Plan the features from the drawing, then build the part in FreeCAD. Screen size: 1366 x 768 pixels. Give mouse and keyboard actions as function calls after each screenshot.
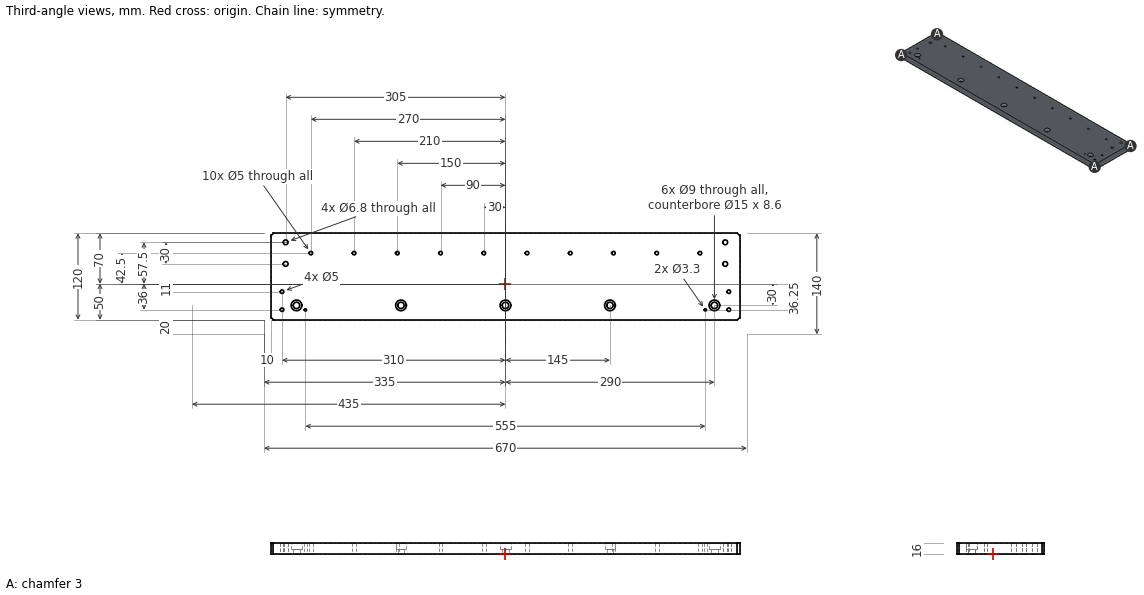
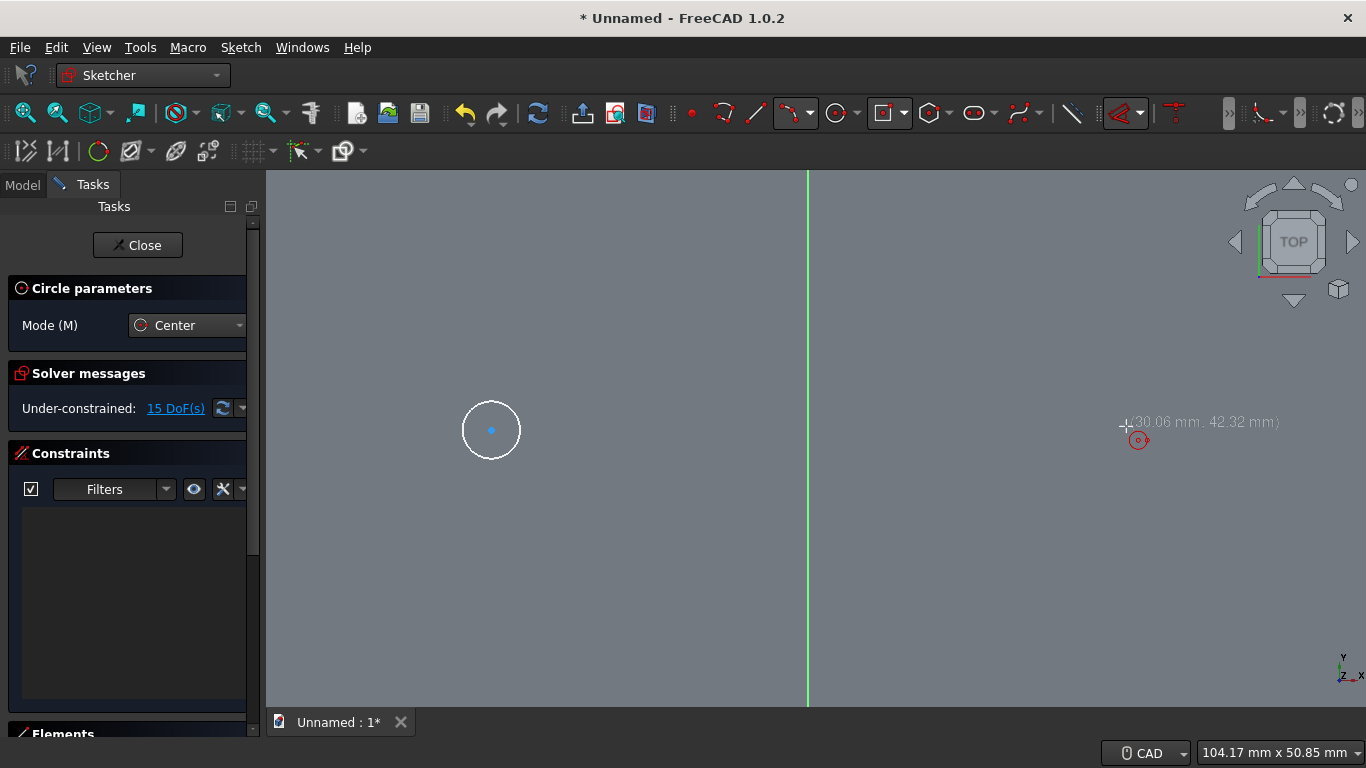
scroll(740, 414, down, 11)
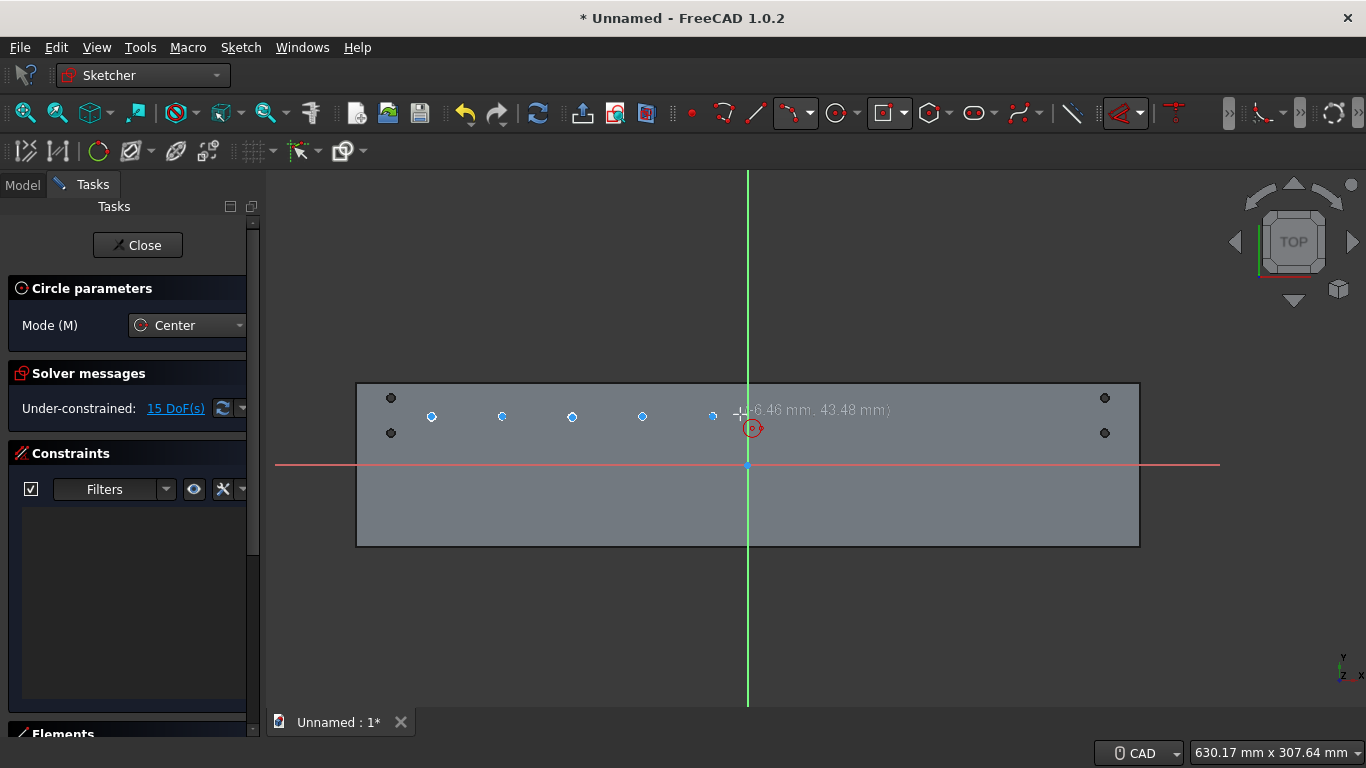
click(783, 416)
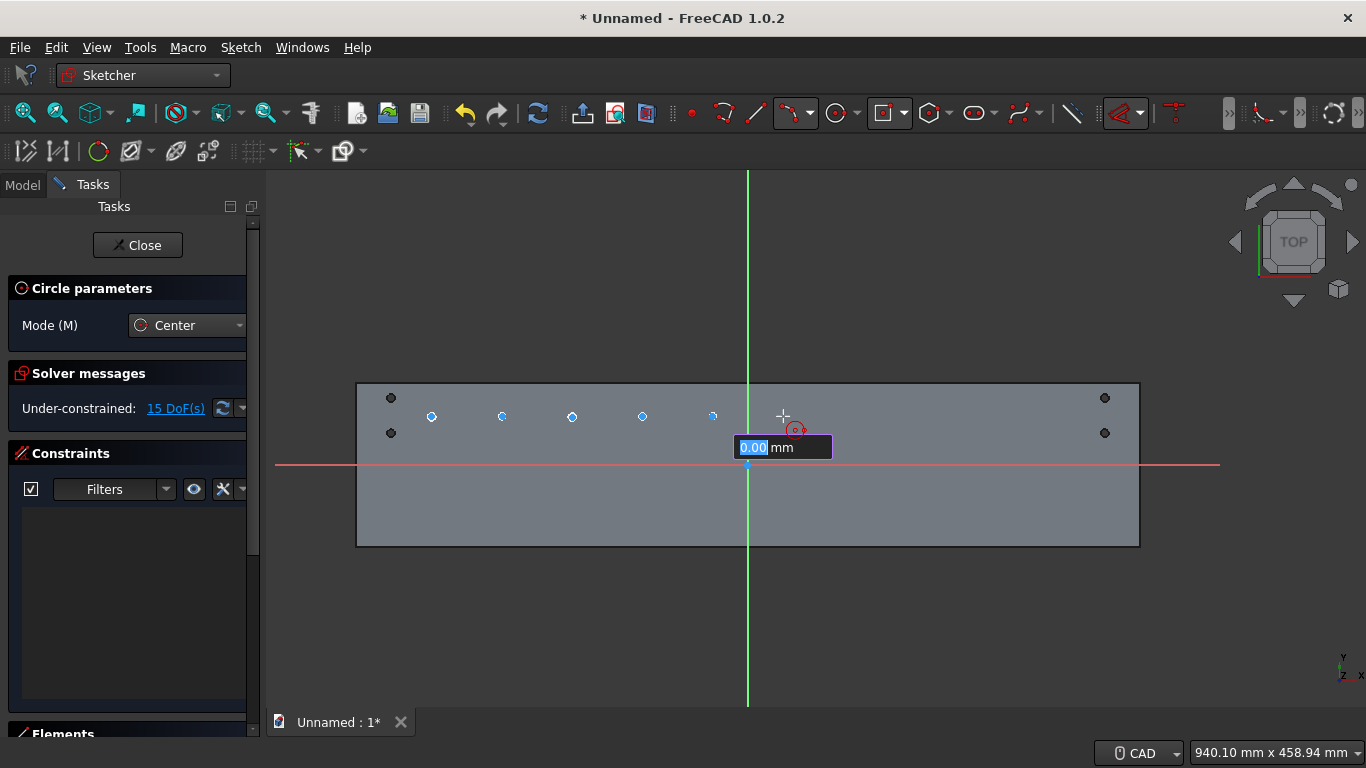
scroll(785, 414, up, 9)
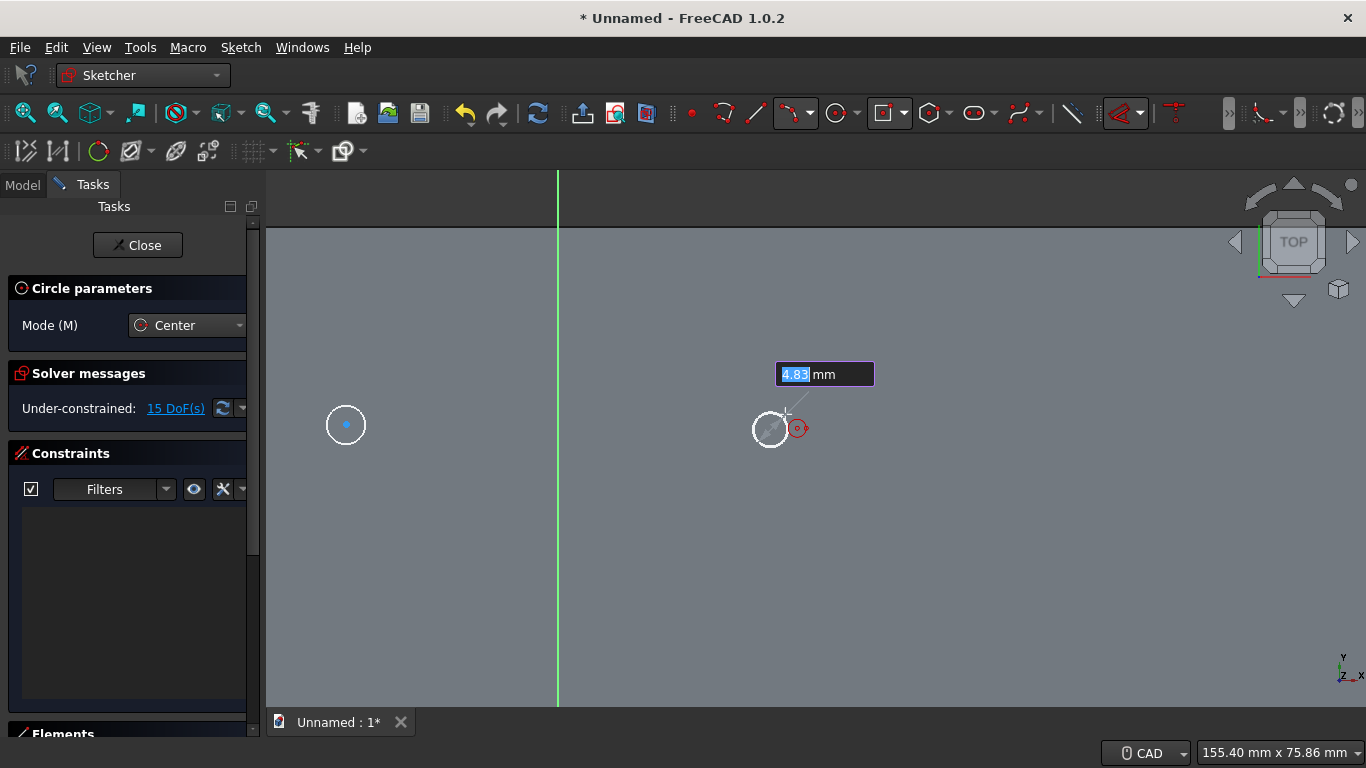
click(783, 409)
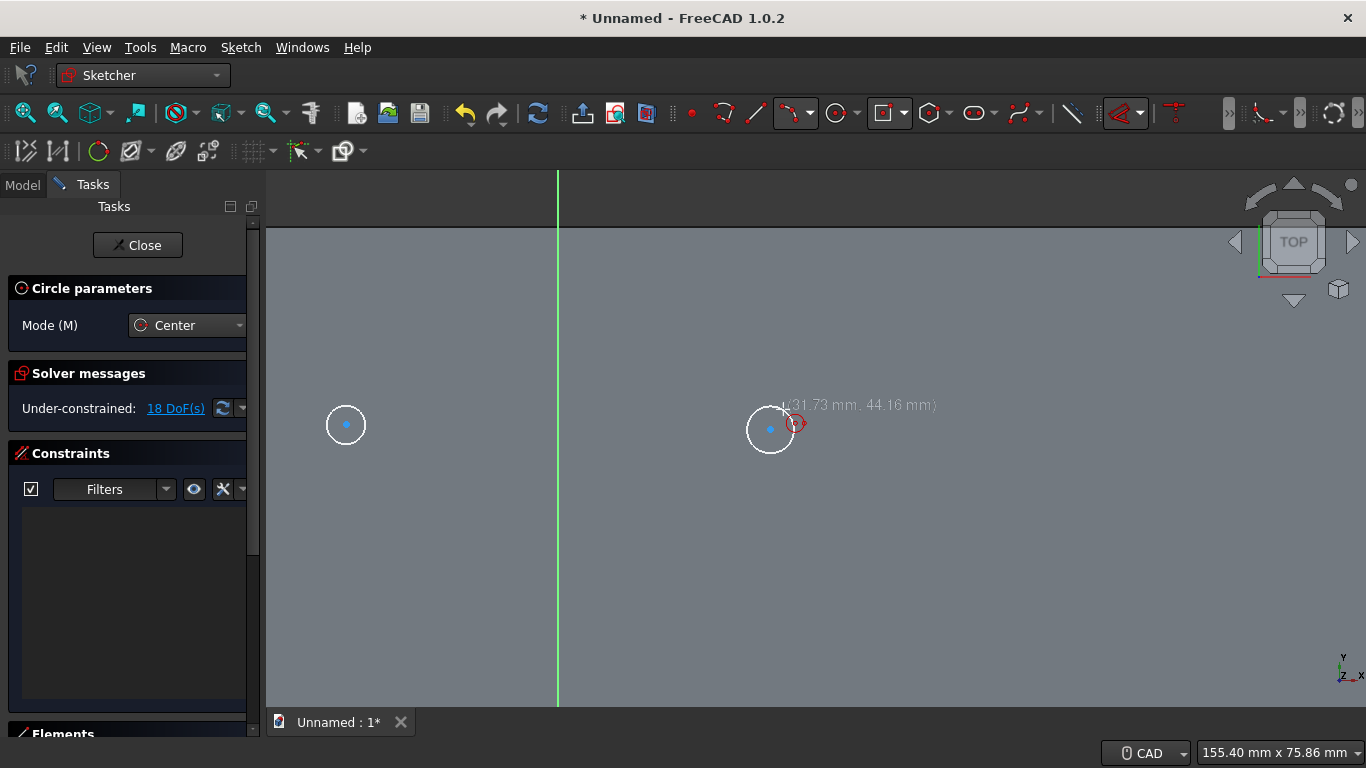
scroll(1195, 422, up, 2)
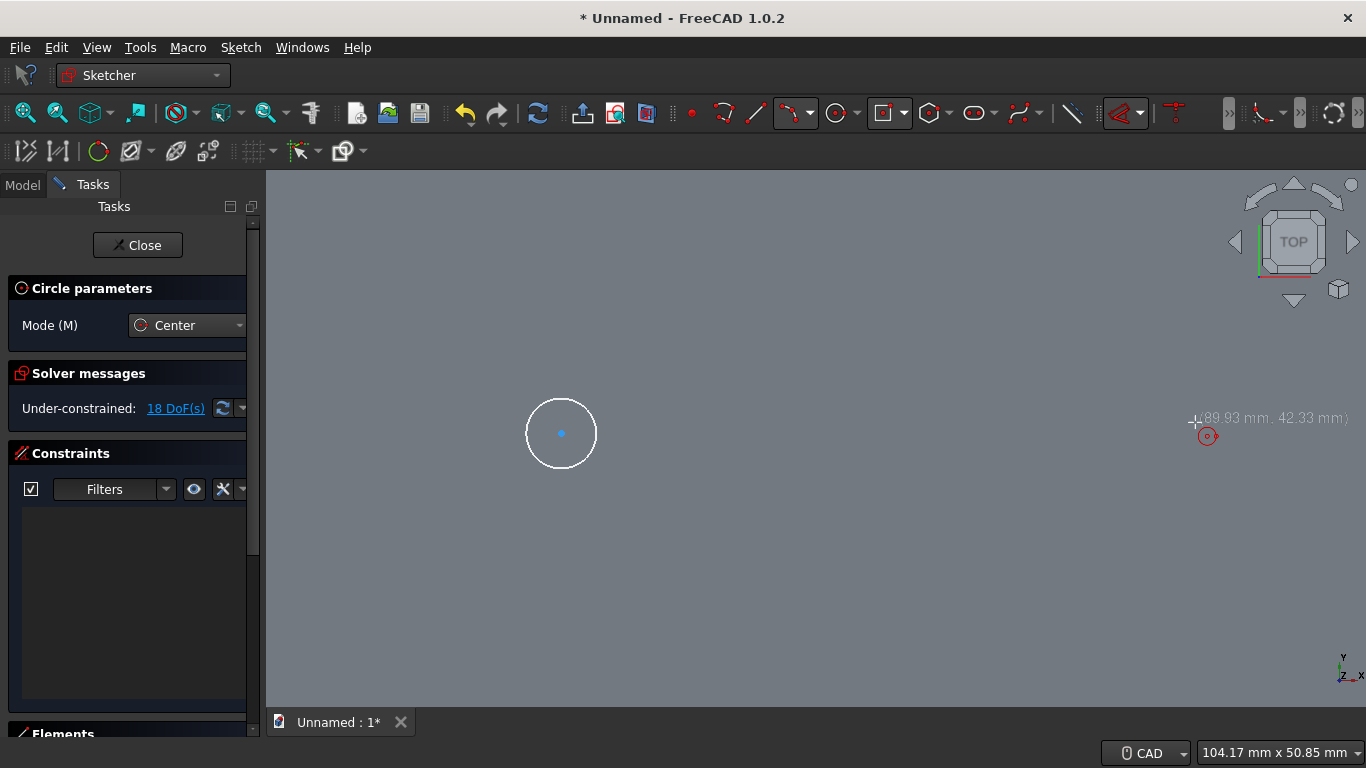
scroll(810, 414, down, 11)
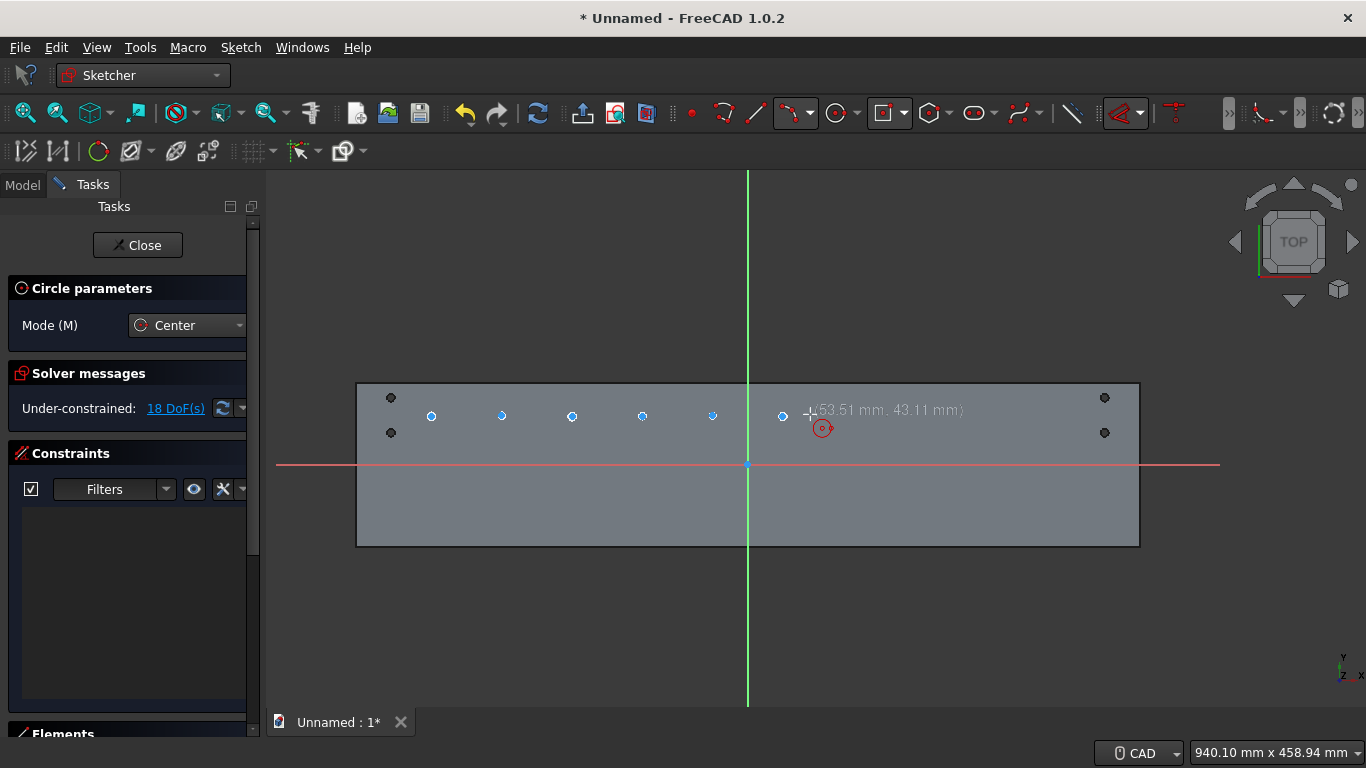
click(853, 415)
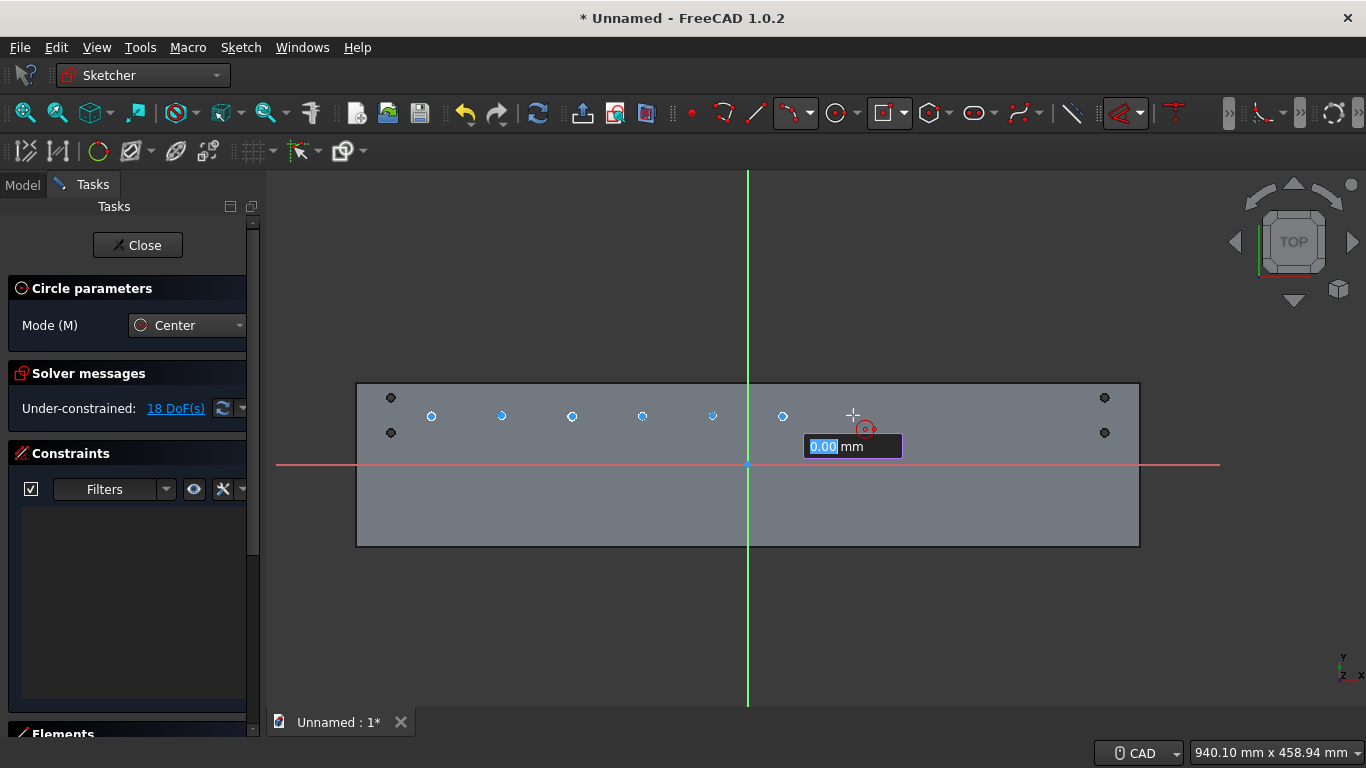
scroll(855, 413, up, 9)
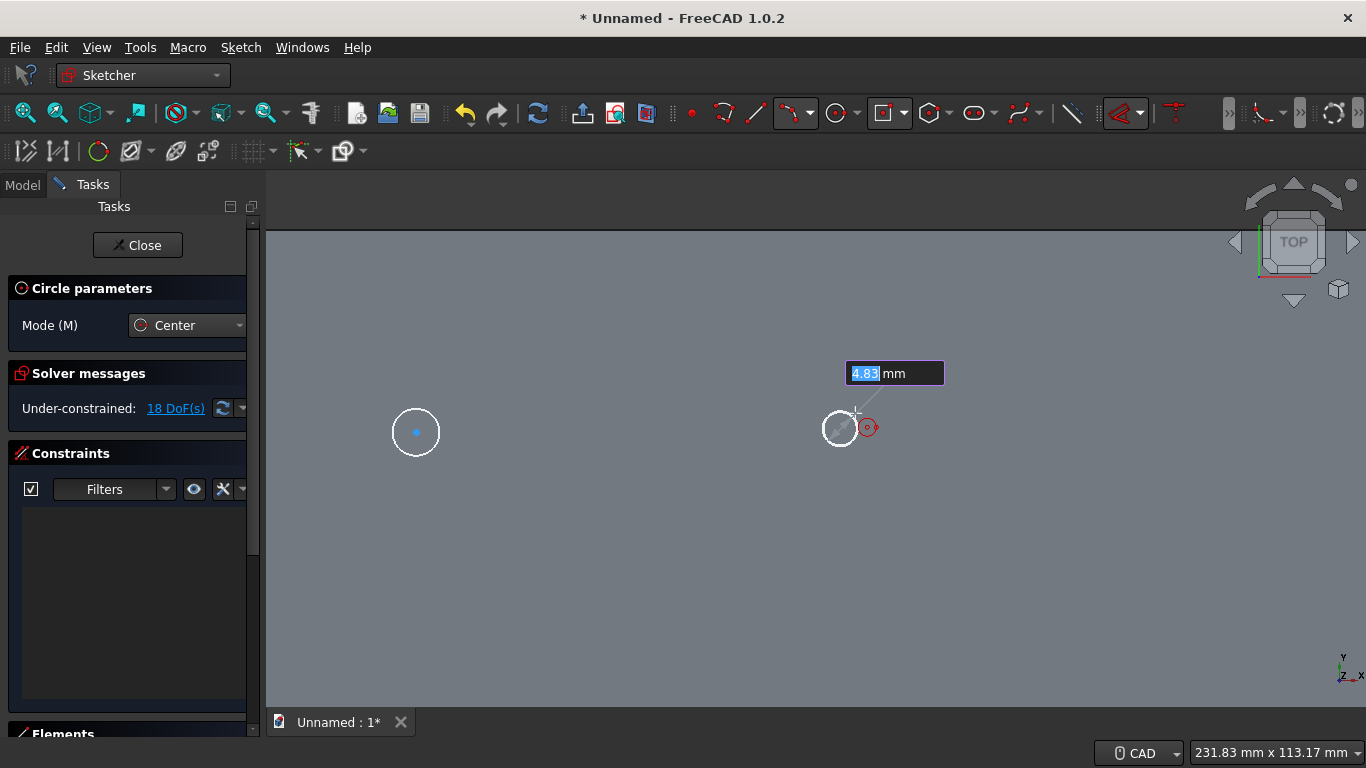
click(854, 412)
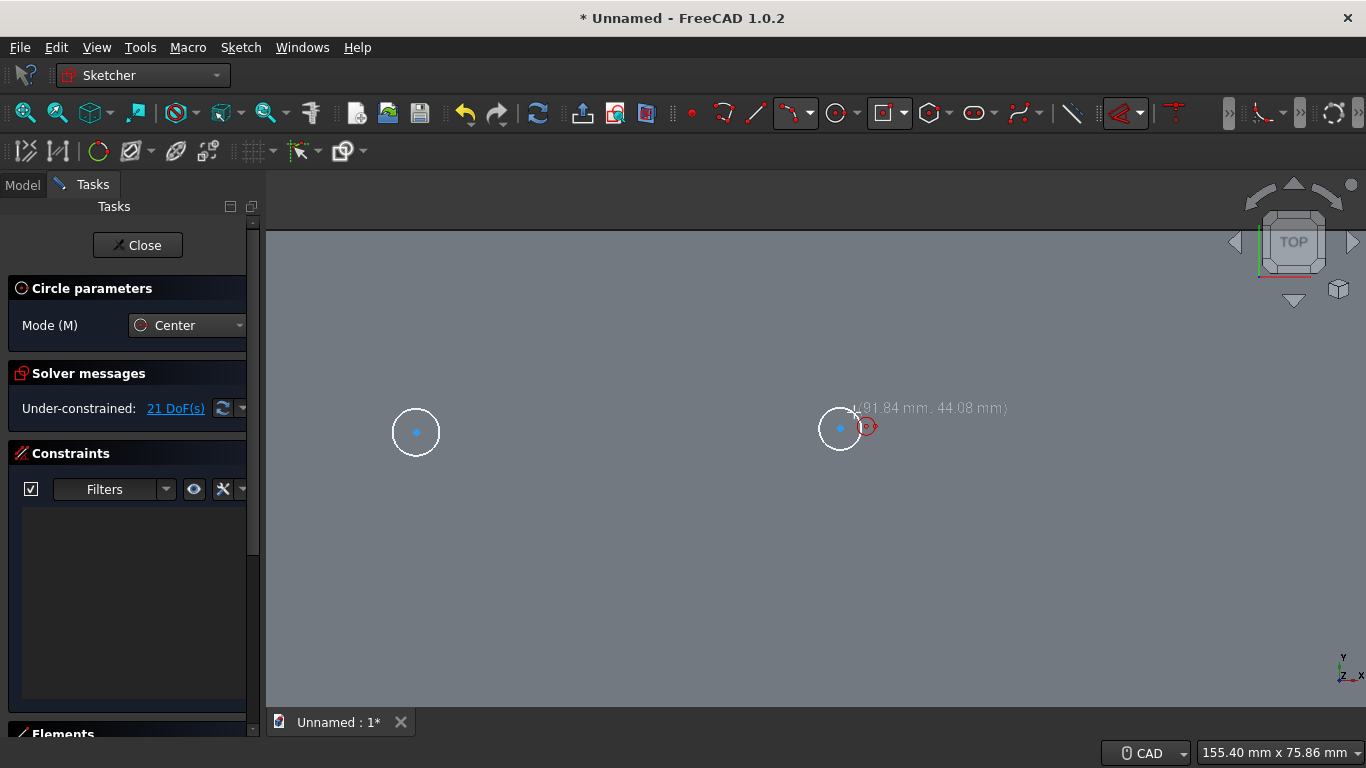
scroll(855, 413, down, 9)